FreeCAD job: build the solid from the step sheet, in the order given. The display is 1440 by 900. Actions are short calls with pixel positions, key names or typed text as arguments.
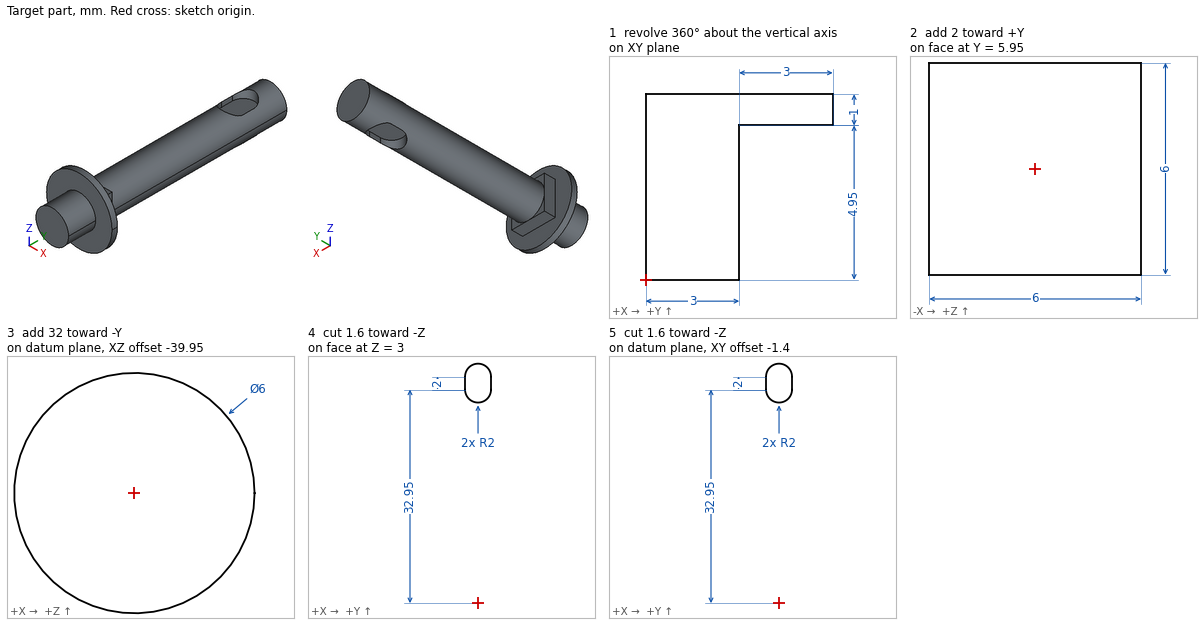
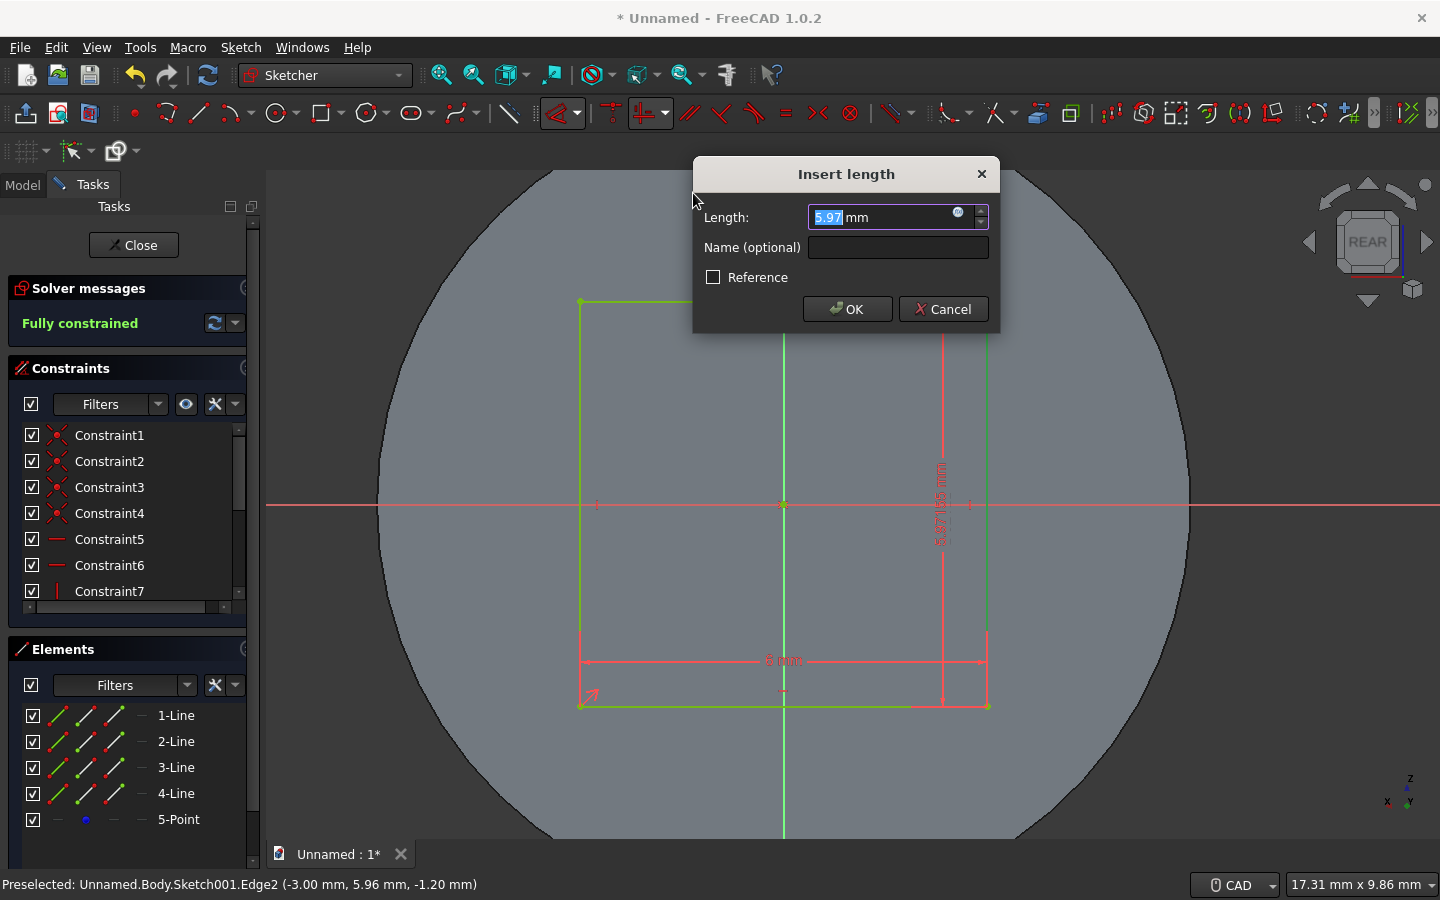
text(6)
key(Return)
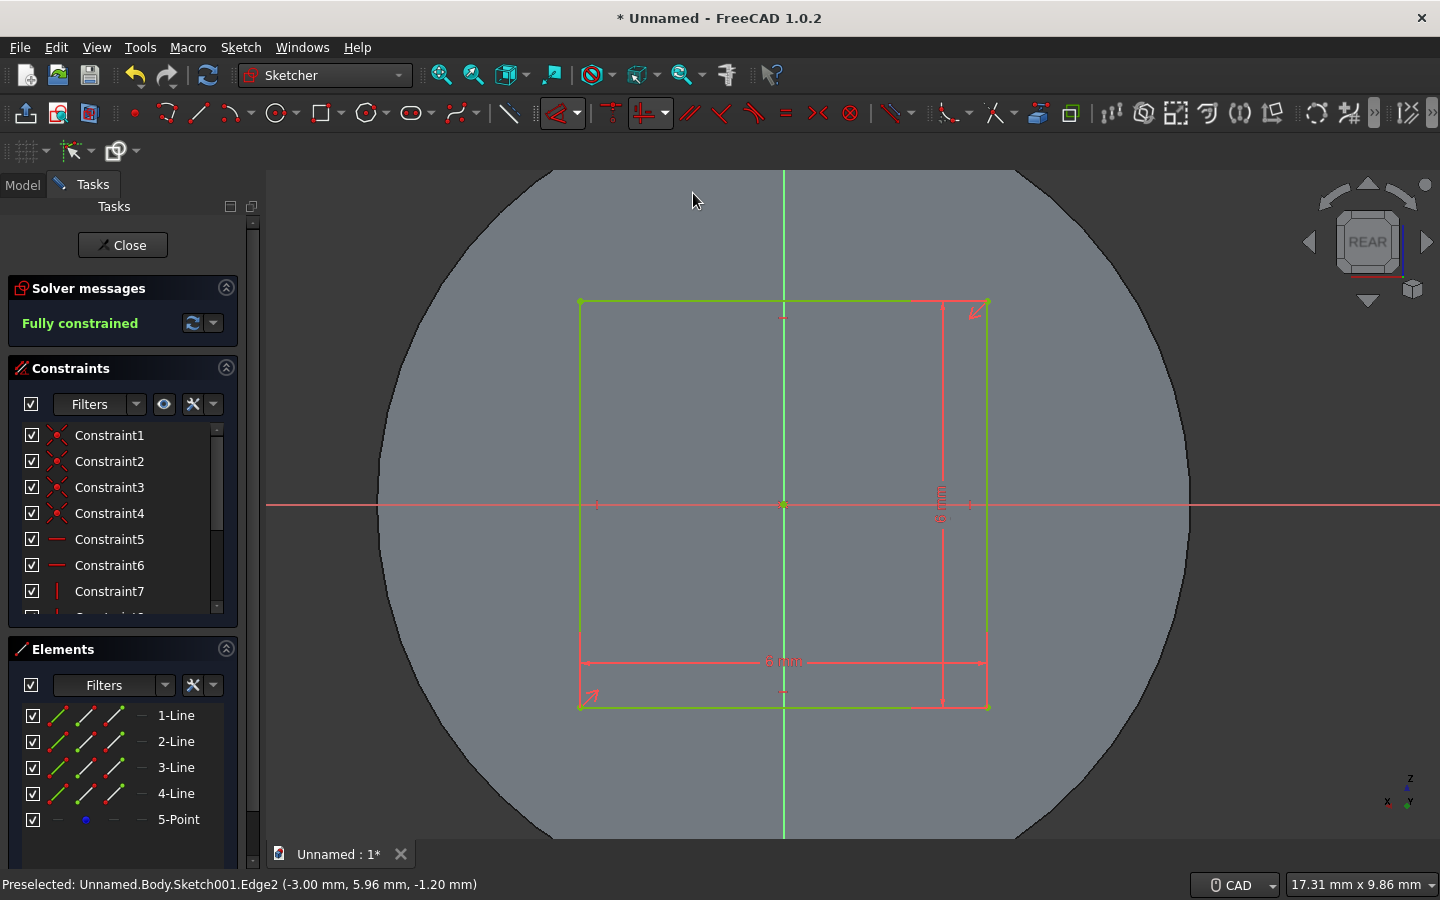
click(123, 245)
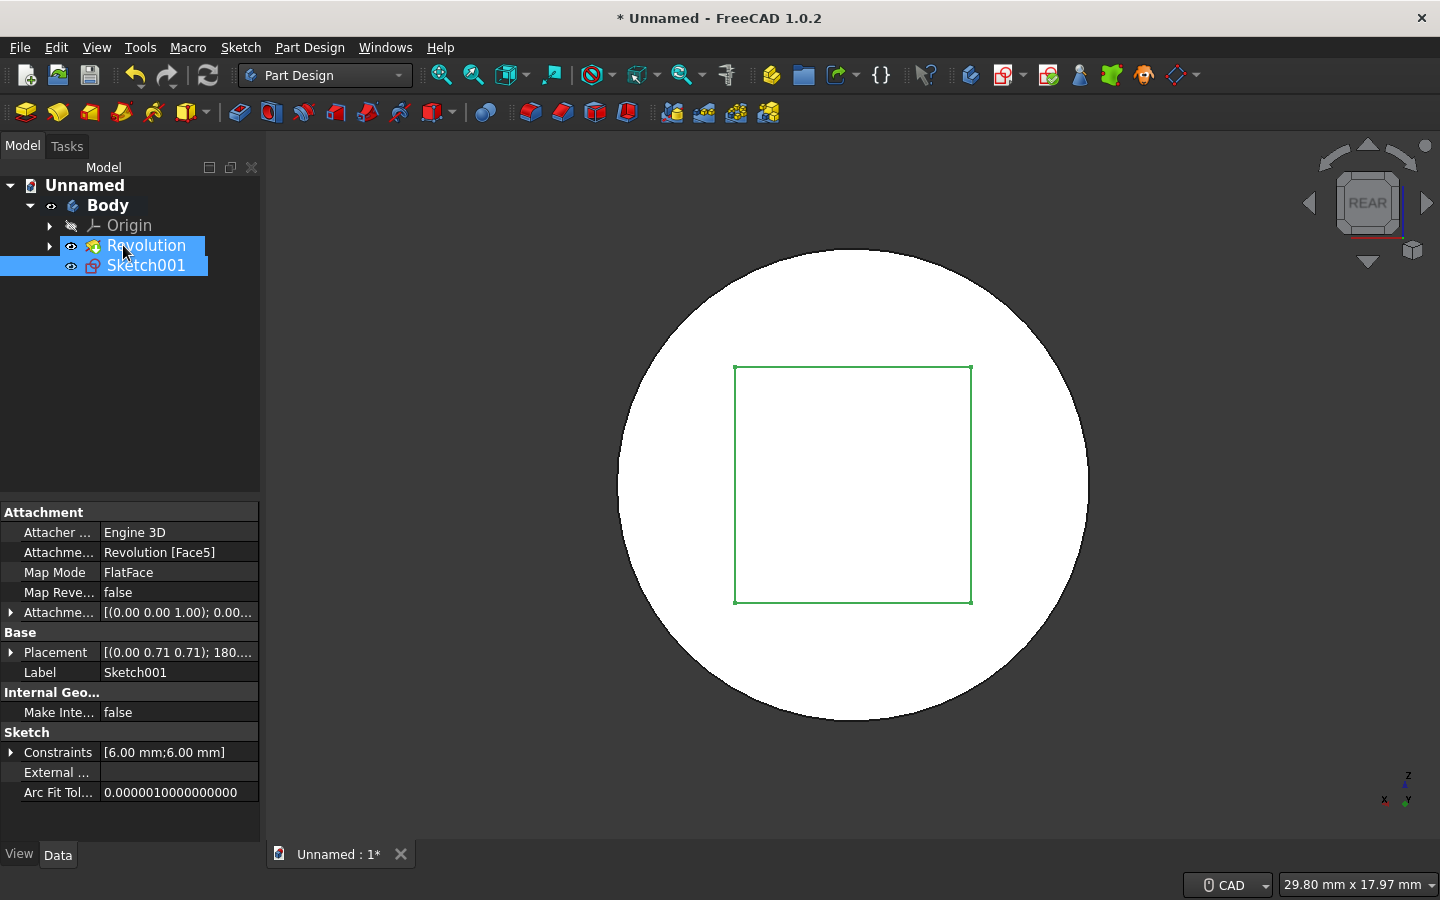
click(26, 112)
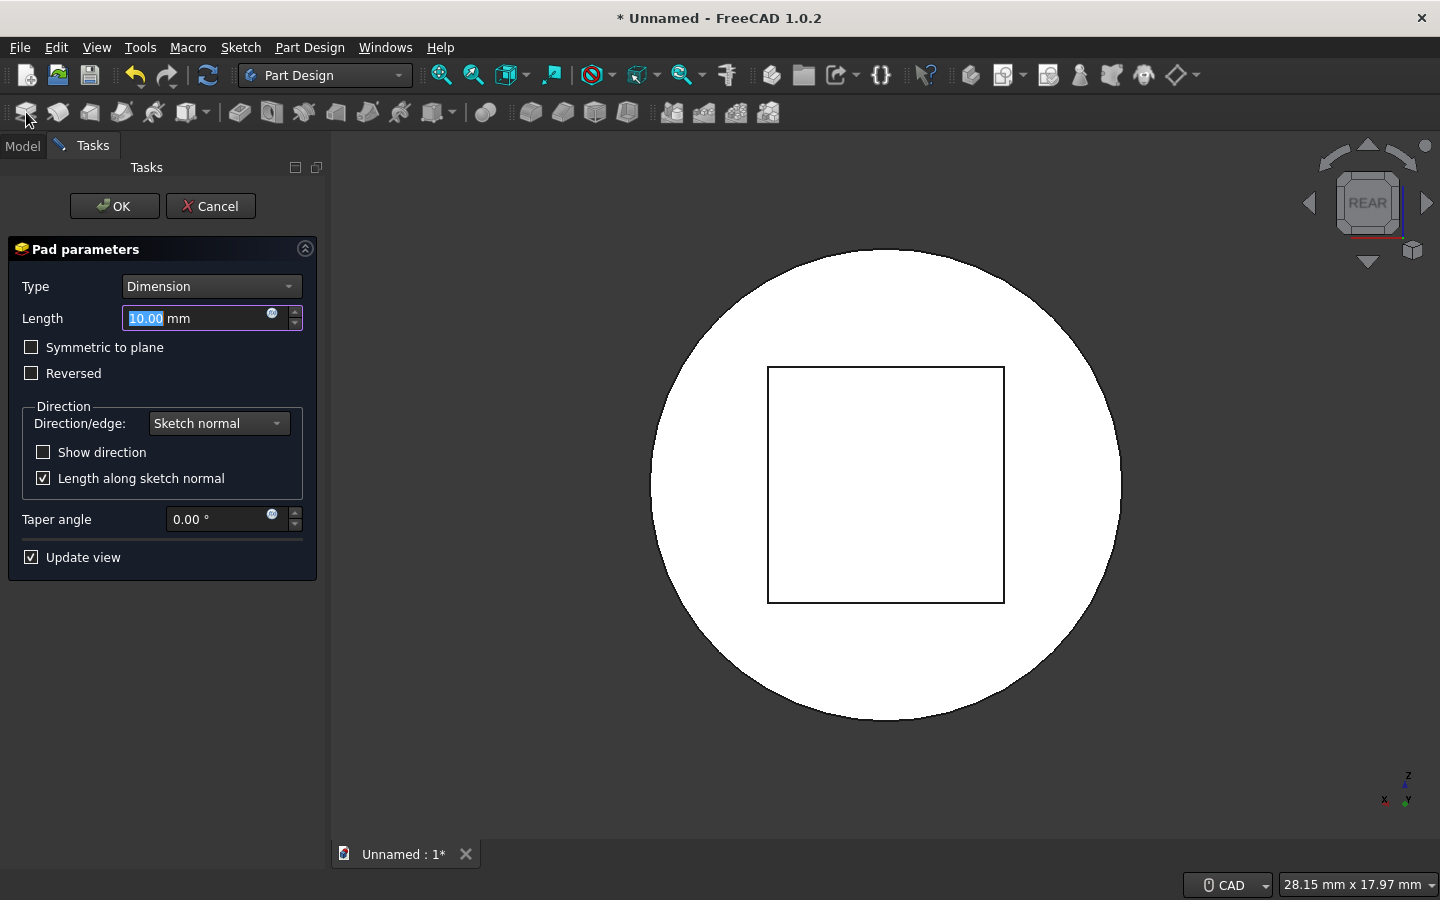
text(2)
key(Tab)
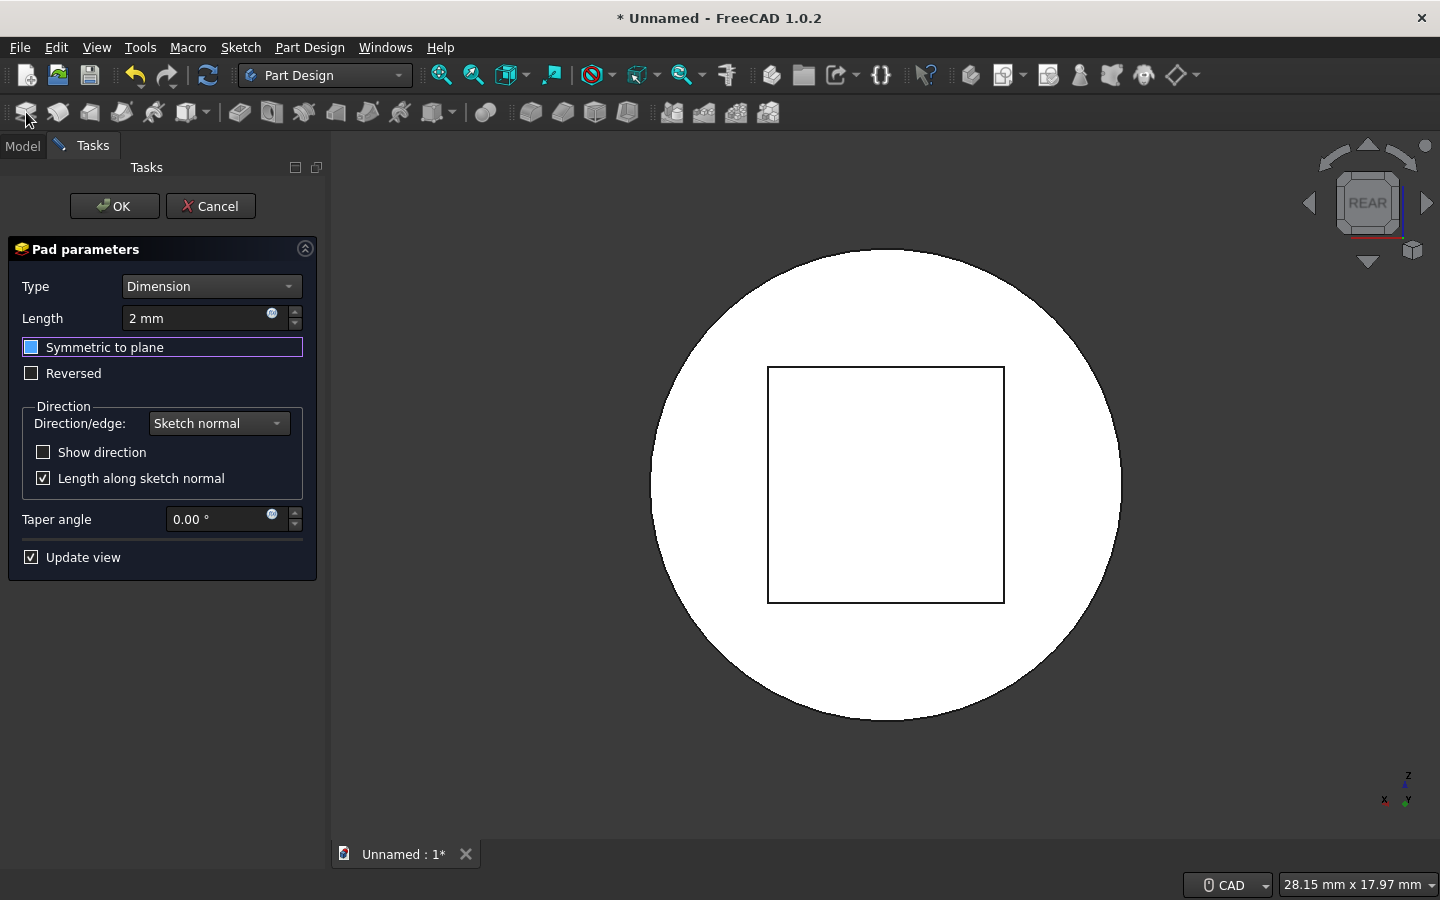
click(115, 206)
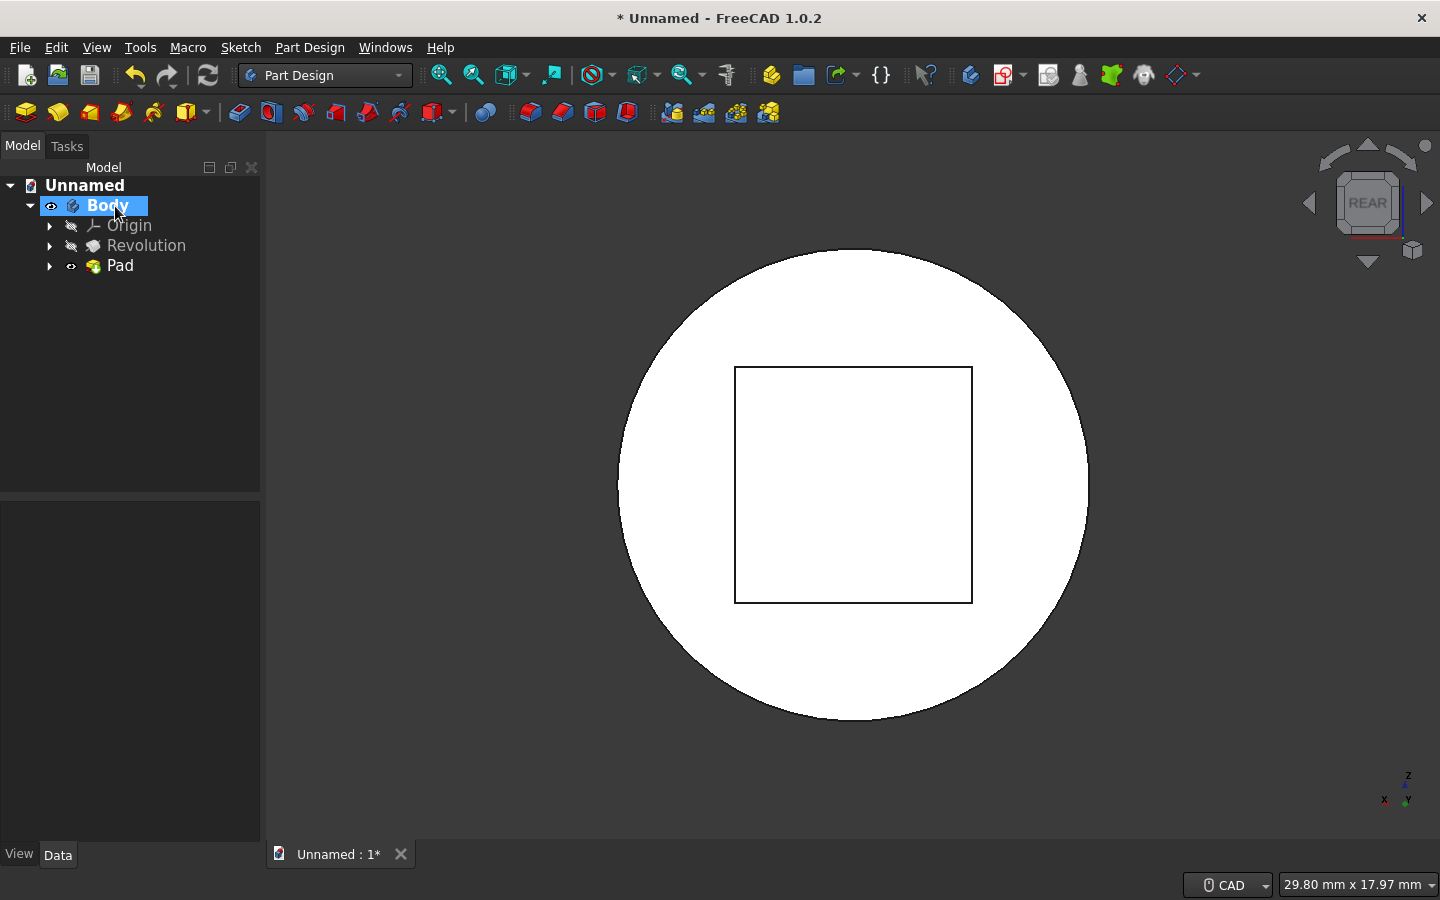
click(50, 226)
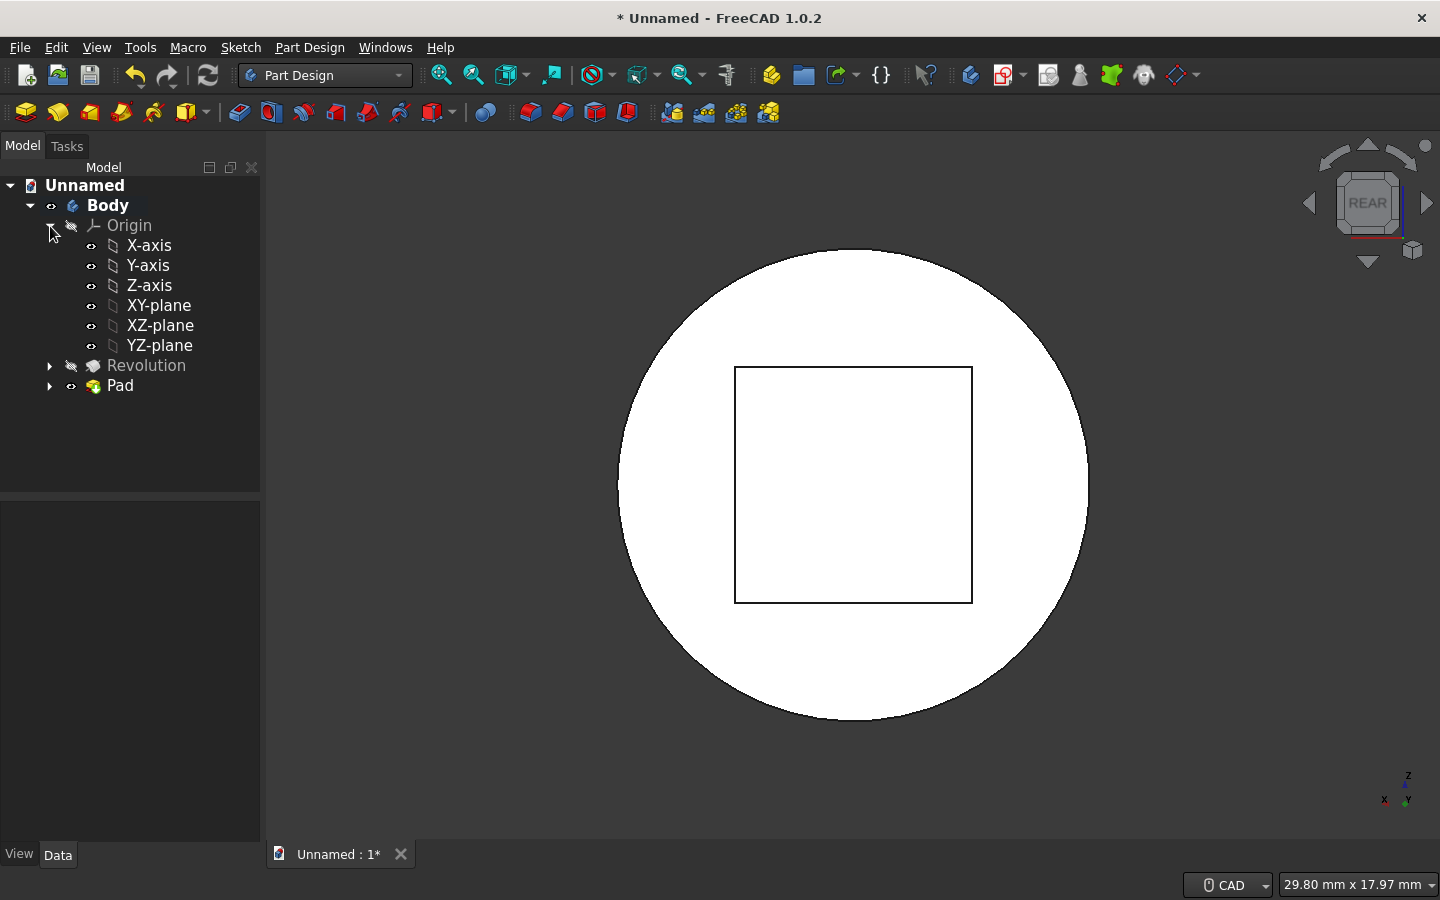
click(136, 326)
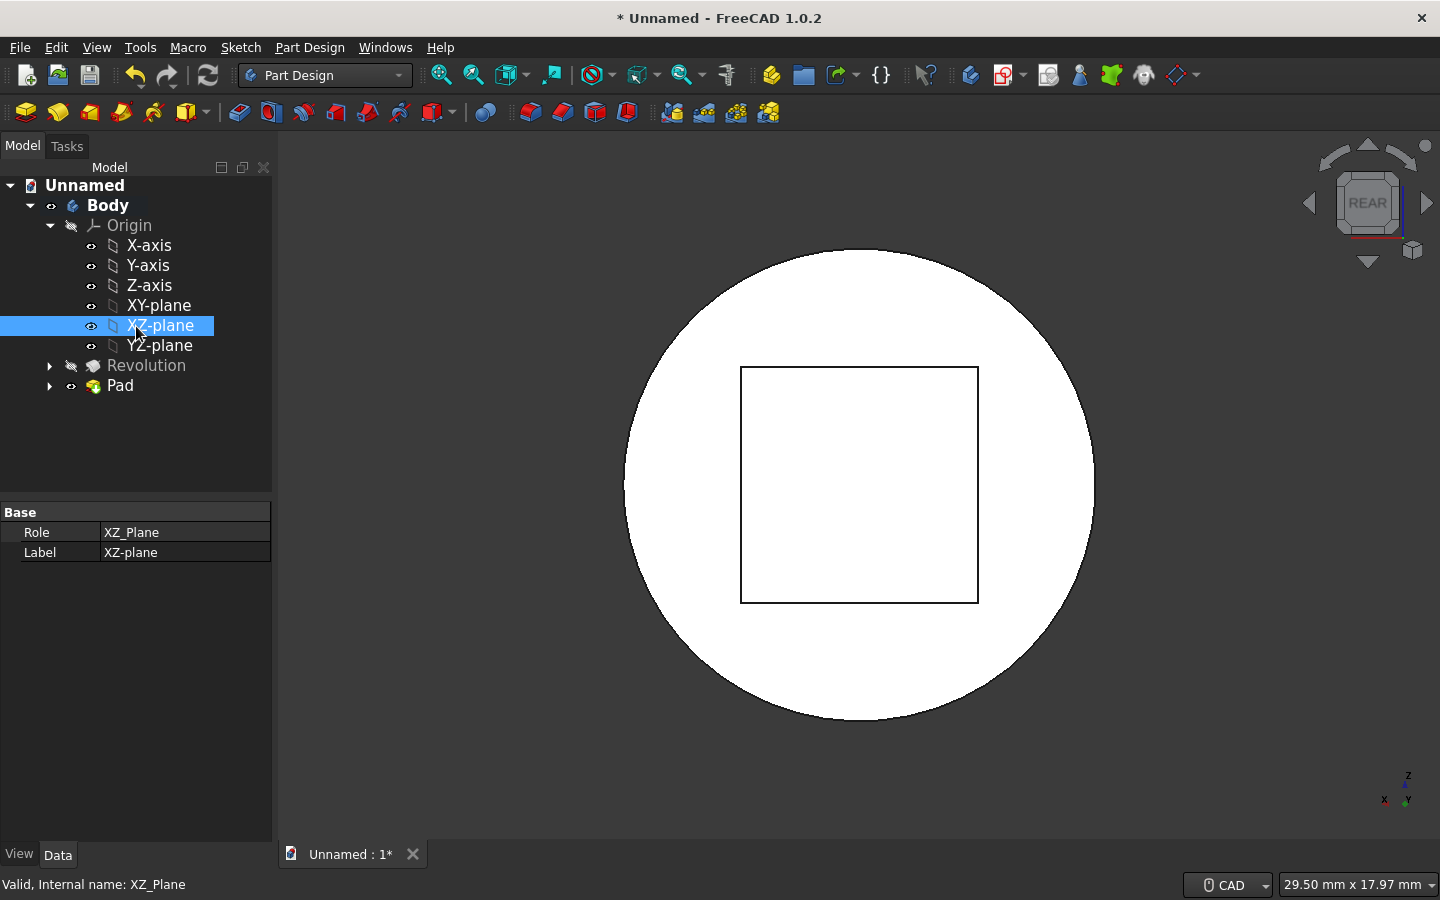
click(1176, 76)